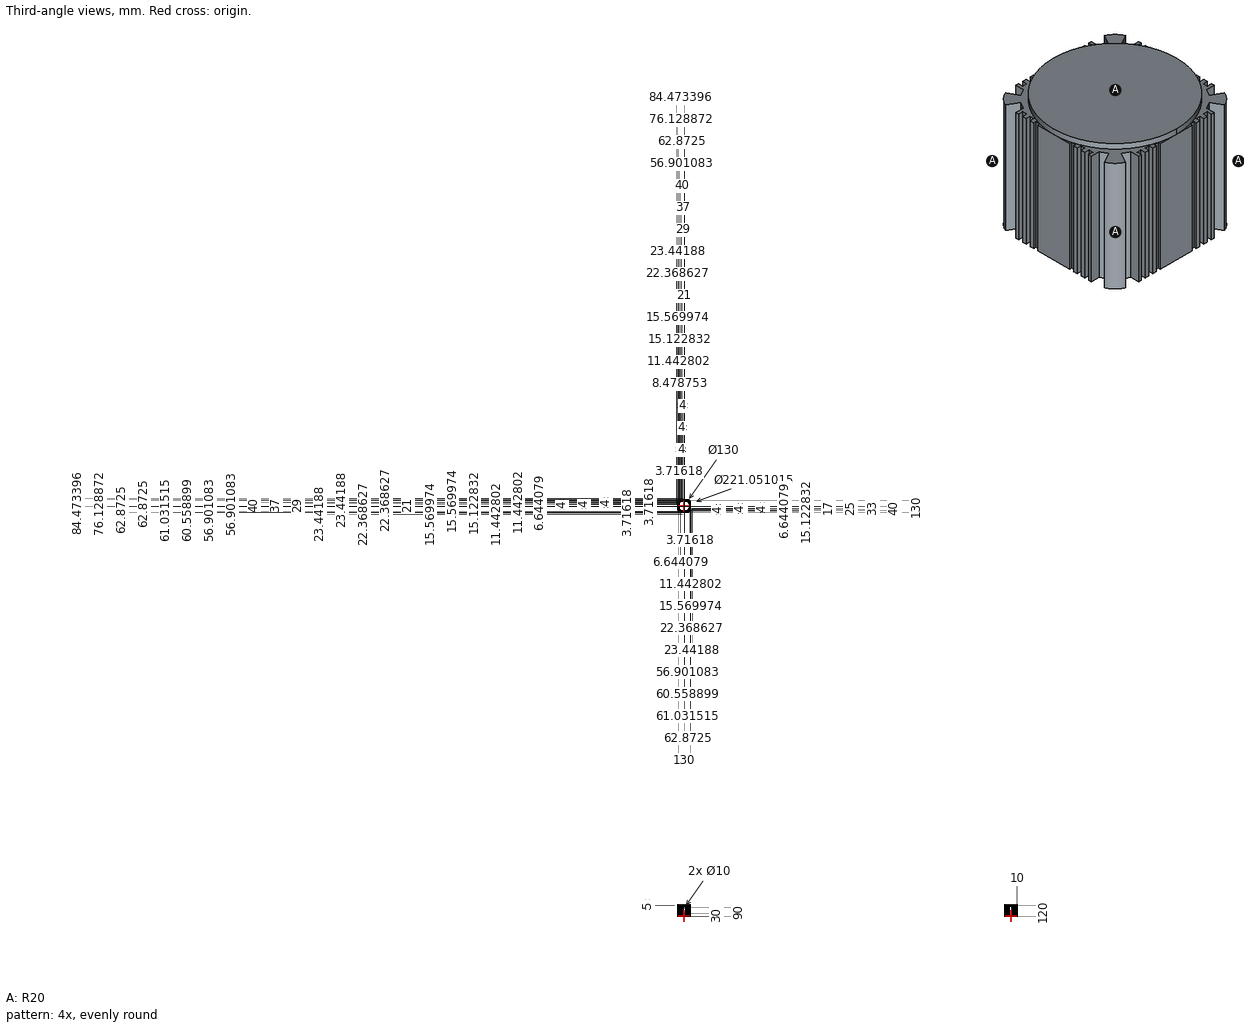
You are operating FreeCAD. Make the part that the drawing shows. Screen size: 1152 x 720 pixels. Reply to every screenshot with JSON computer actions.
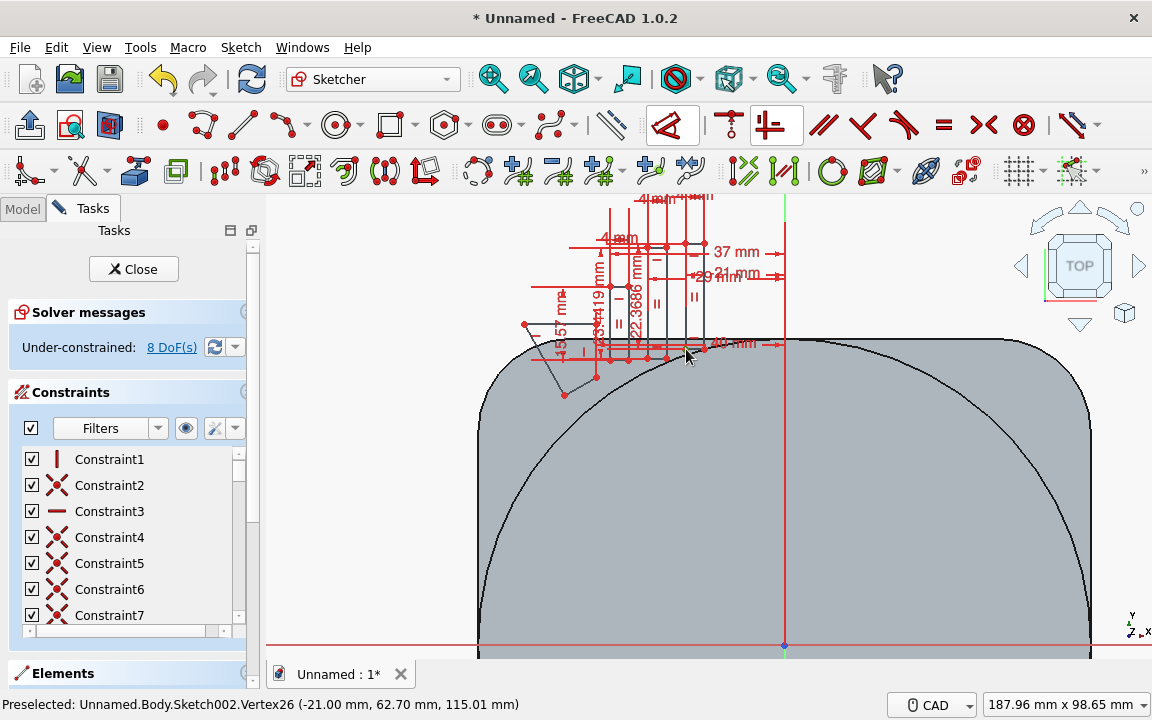
{"action": "left_click", "coordinate": [694, 126]}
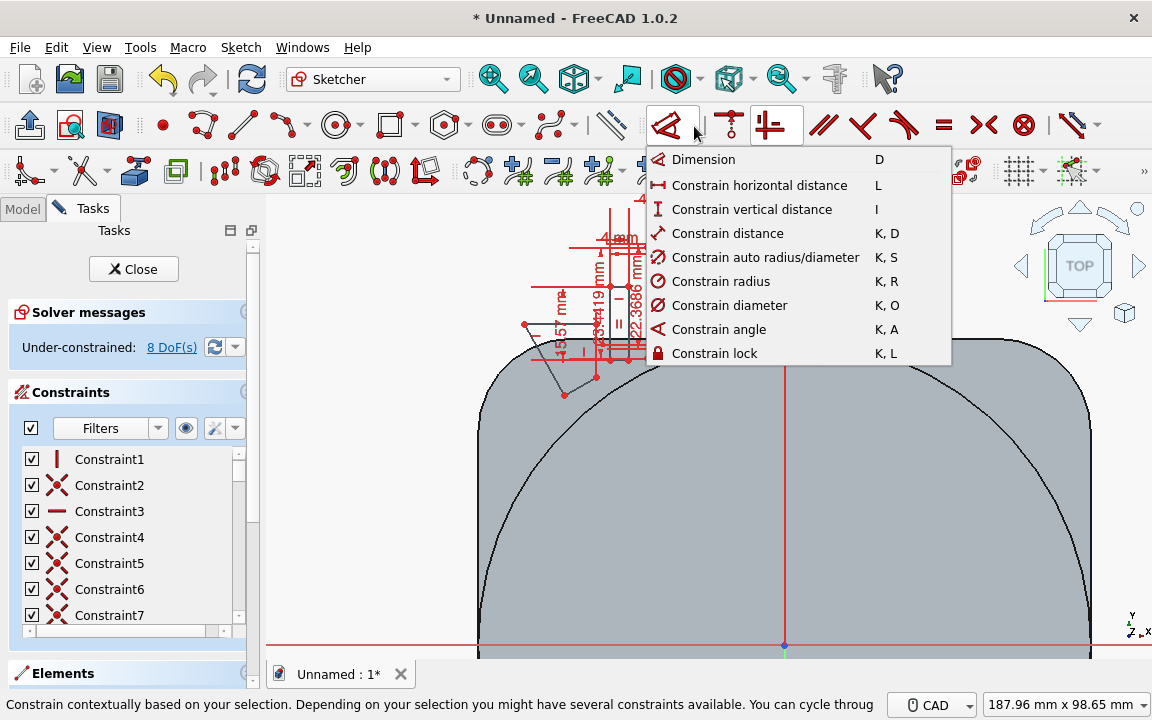
{"action": "left_click", "coordinate": [799, 209]}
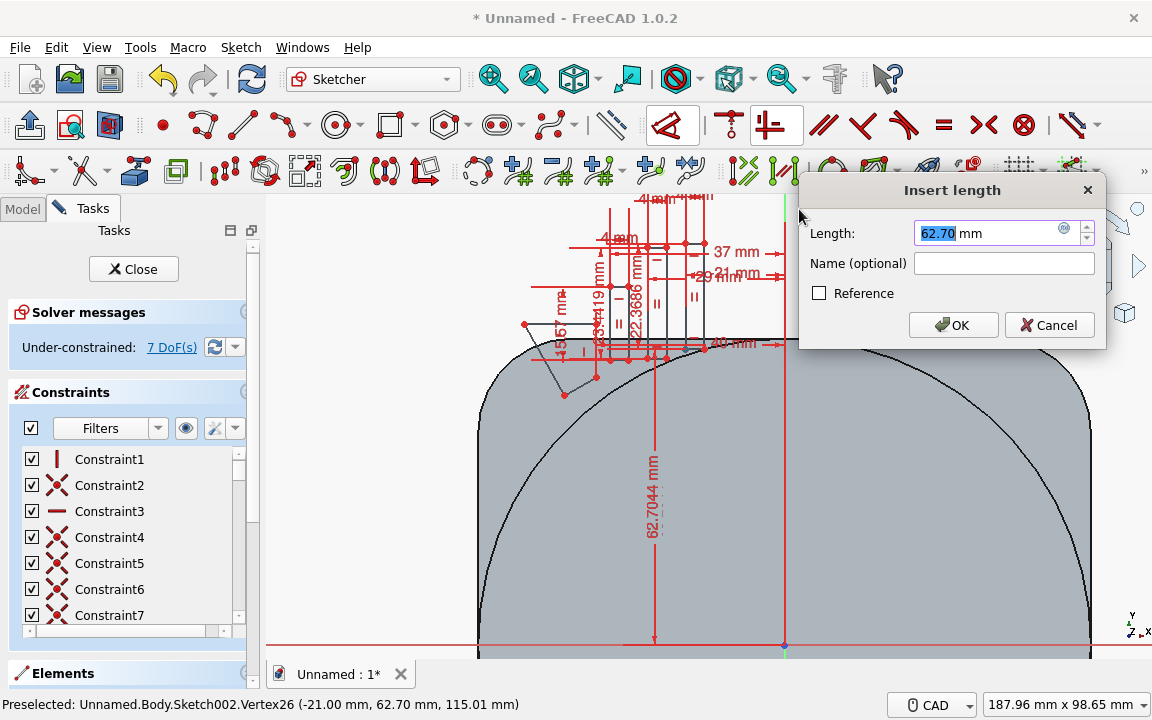
{"action": "type", "text": "62.8725"}
{"action": "key", "text": "Return"}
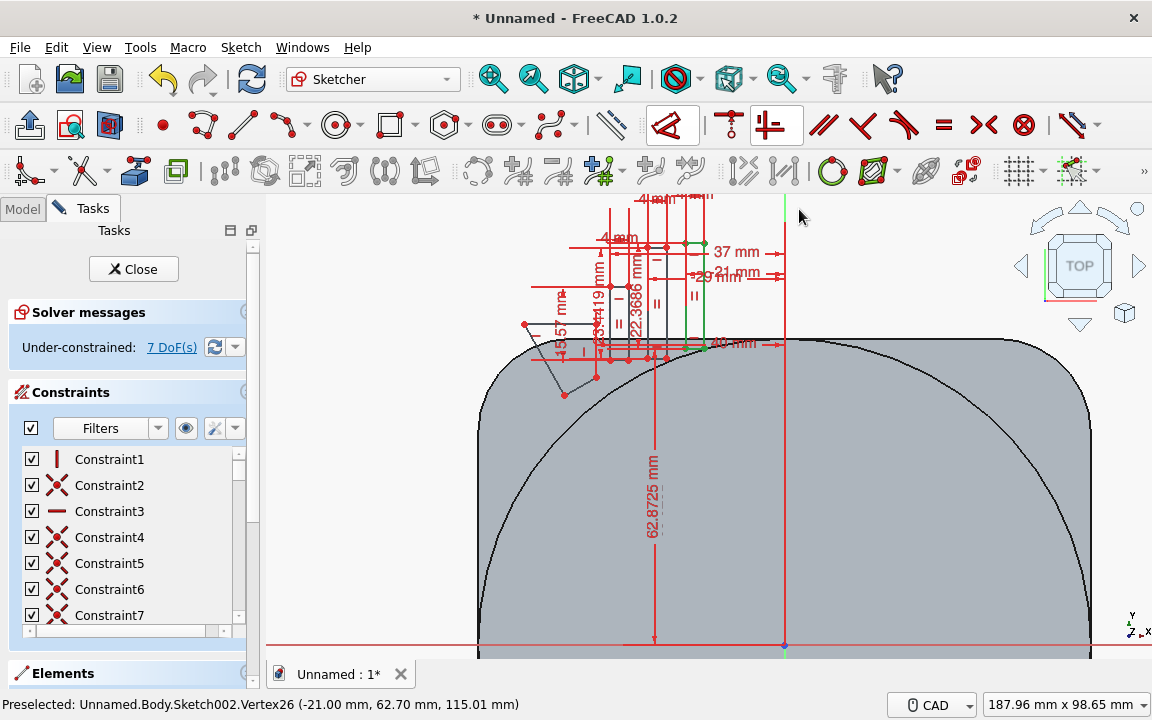
{"action": "scroll", "coordinate": [574, 390], "scroll_direction": "up", "scroll_amount": 5}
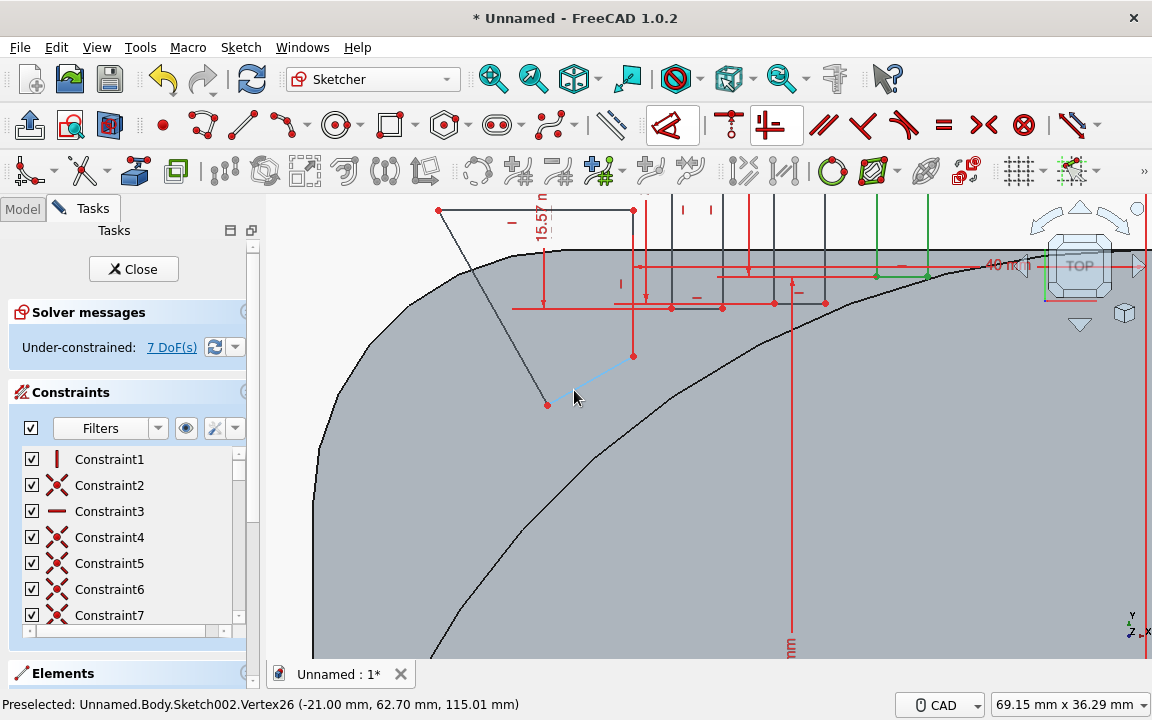
{"action": "left_click", "coordinate": [573, 390]}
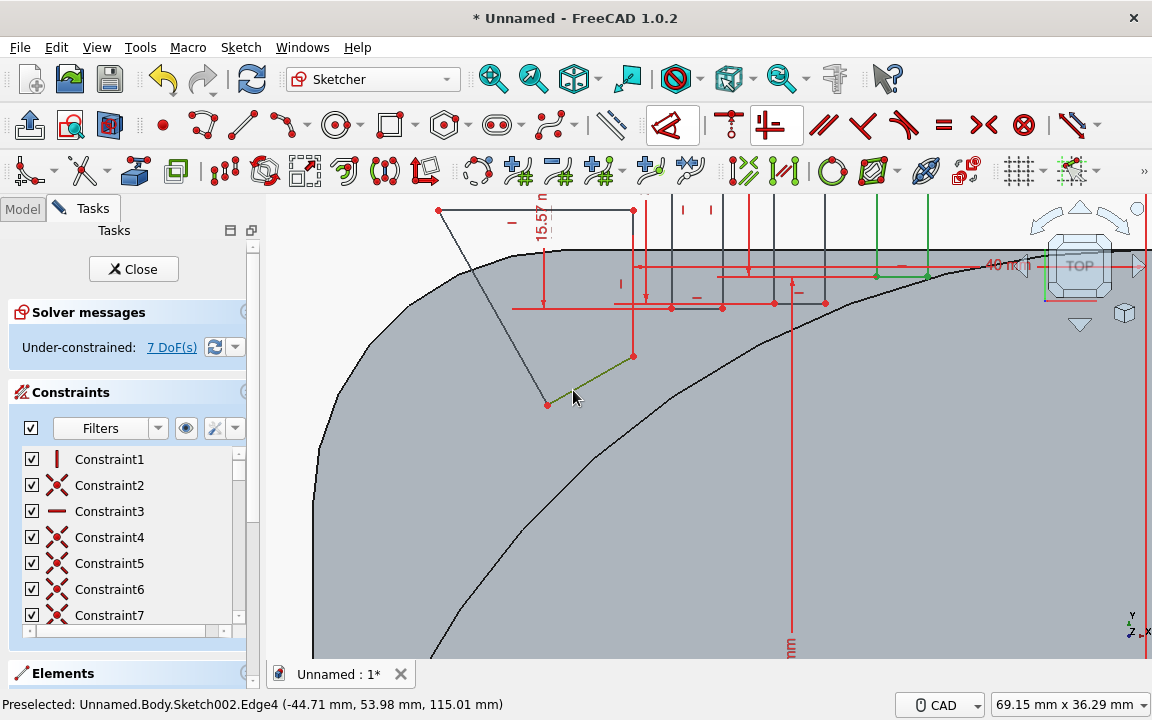
{"action": "key", "text": "i"}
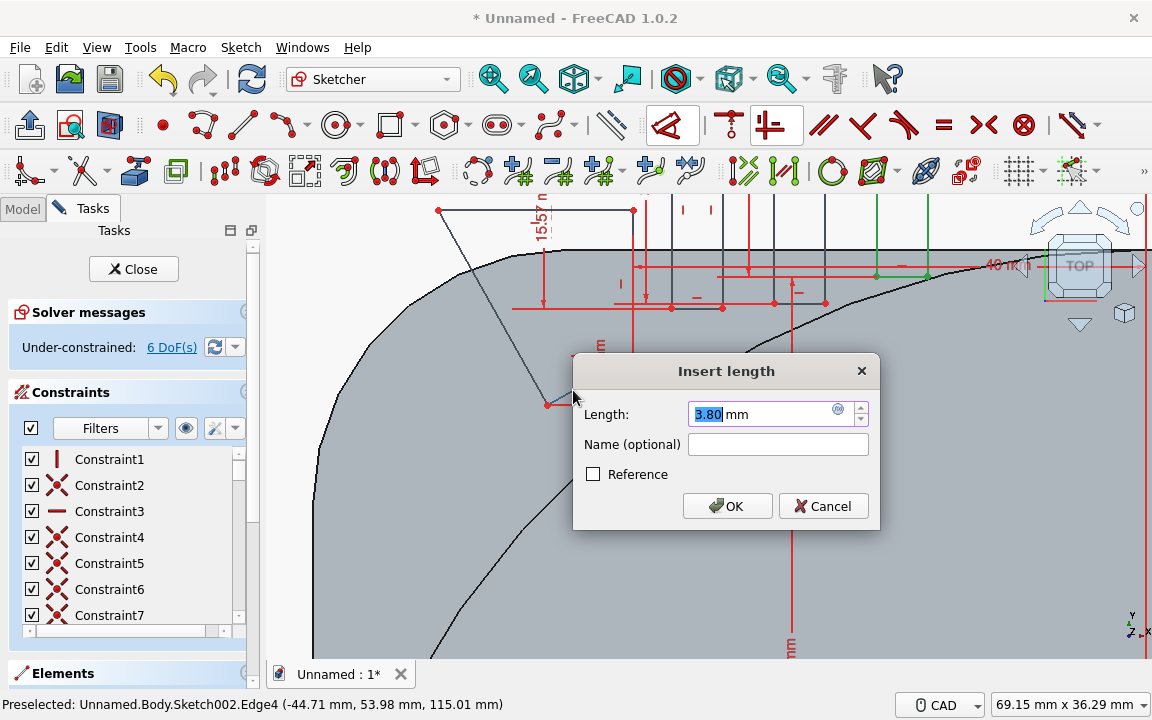
{"action": "type", "text": "3.71618"}
{"action": "key", "text": "Return"}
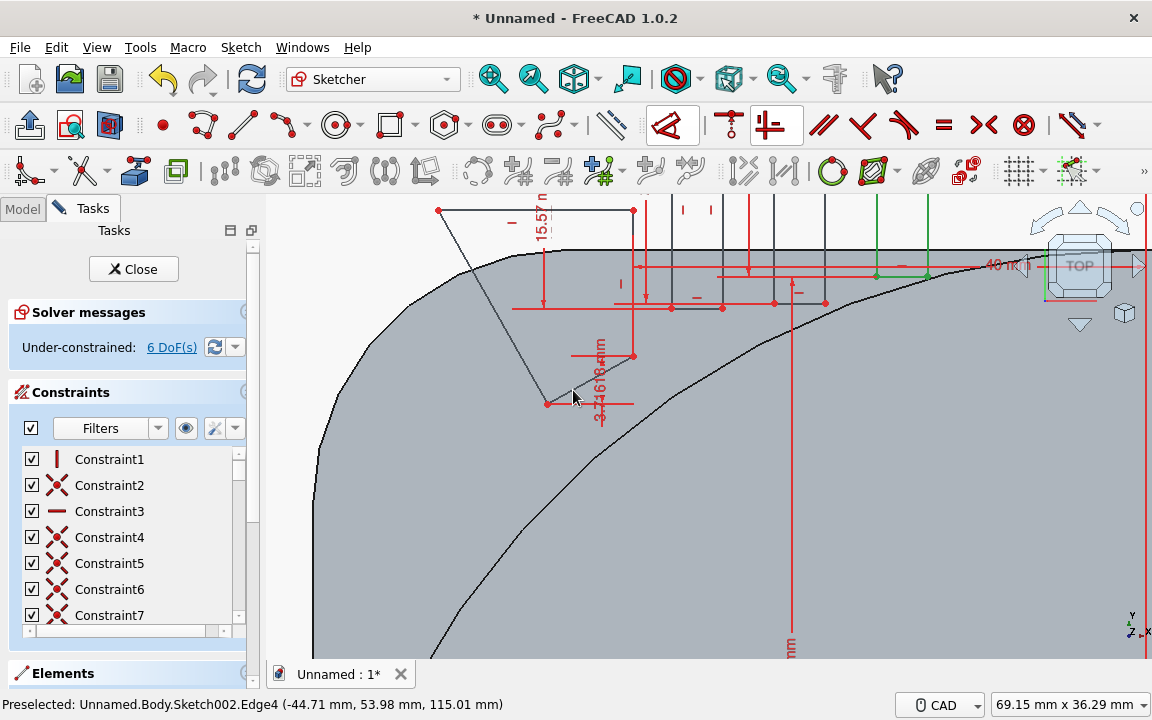
{"action": "left_click", "coordinate": [633, 313]}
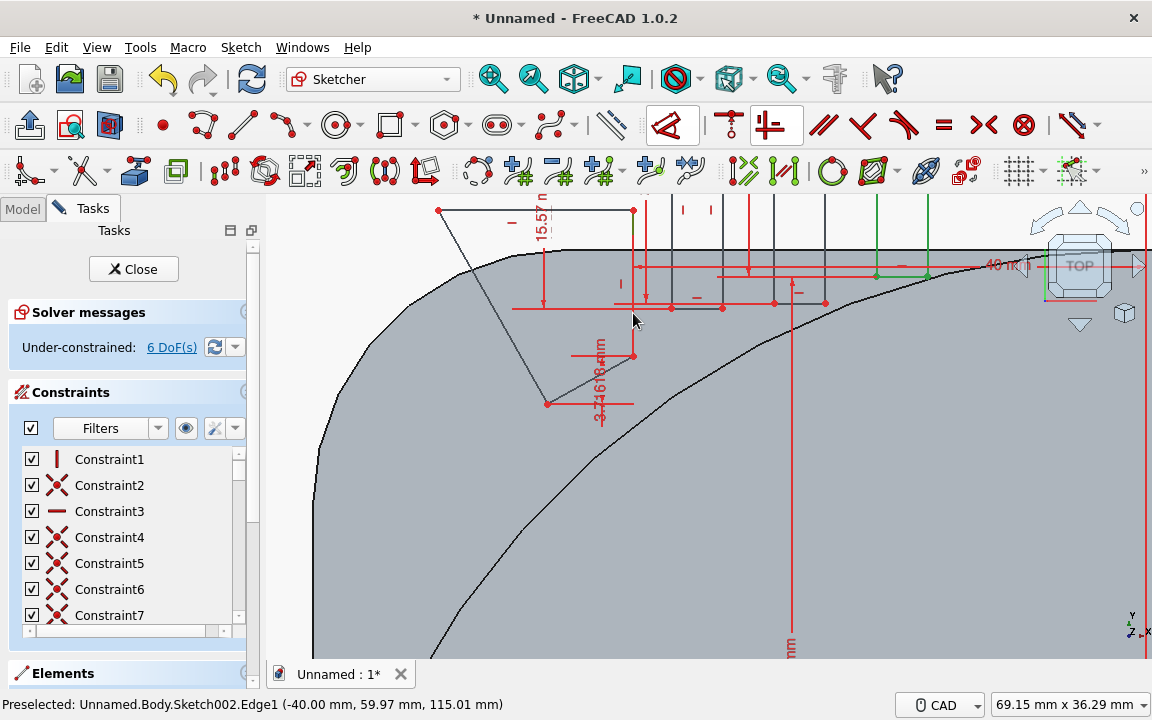
{"action": "key", "text": "i"}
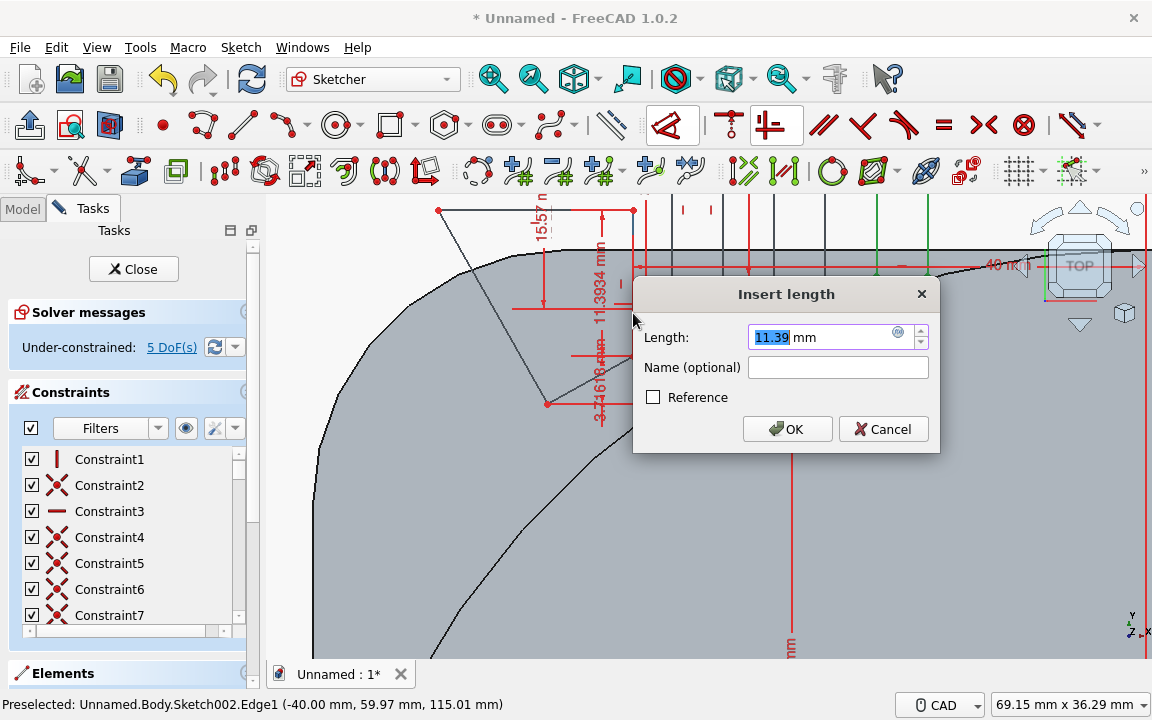
{"action": "type", "text": "11.442802"}
{"action": "key", "text": "Return"}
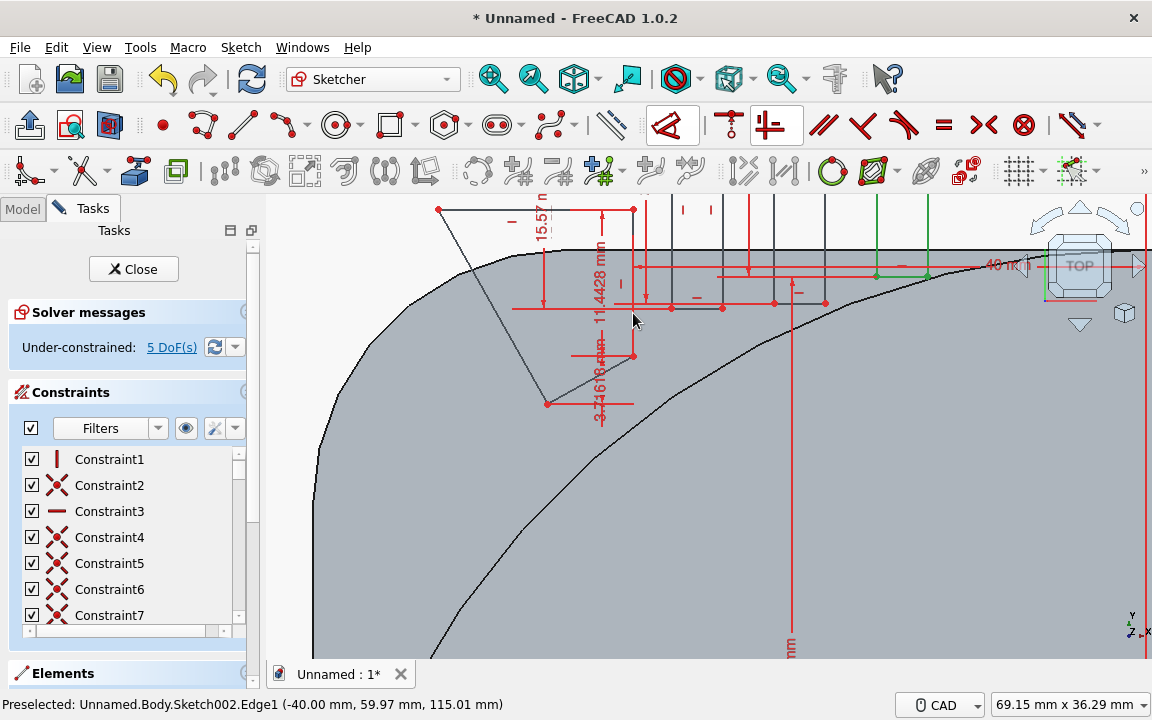
{"action": "scroll", "coordinate": [591, 391], "scroll_direction": "down", "scroll_amount": 7}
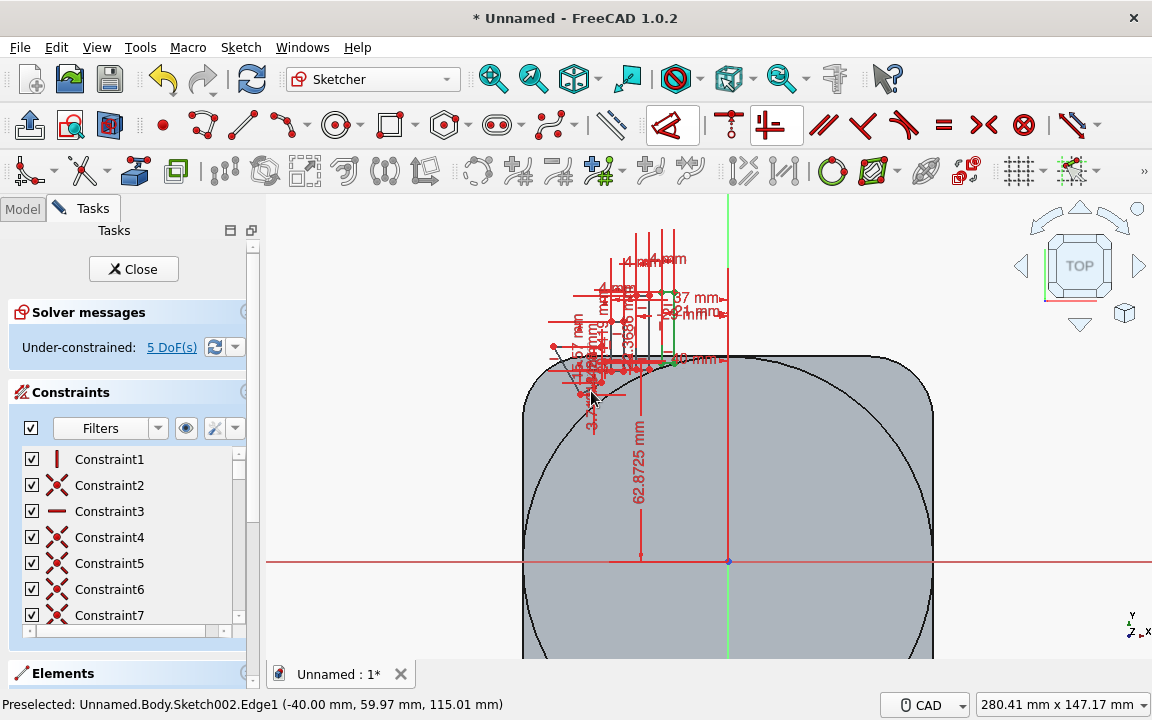
{"action": "left_click", "coordinate": [568, 347]}